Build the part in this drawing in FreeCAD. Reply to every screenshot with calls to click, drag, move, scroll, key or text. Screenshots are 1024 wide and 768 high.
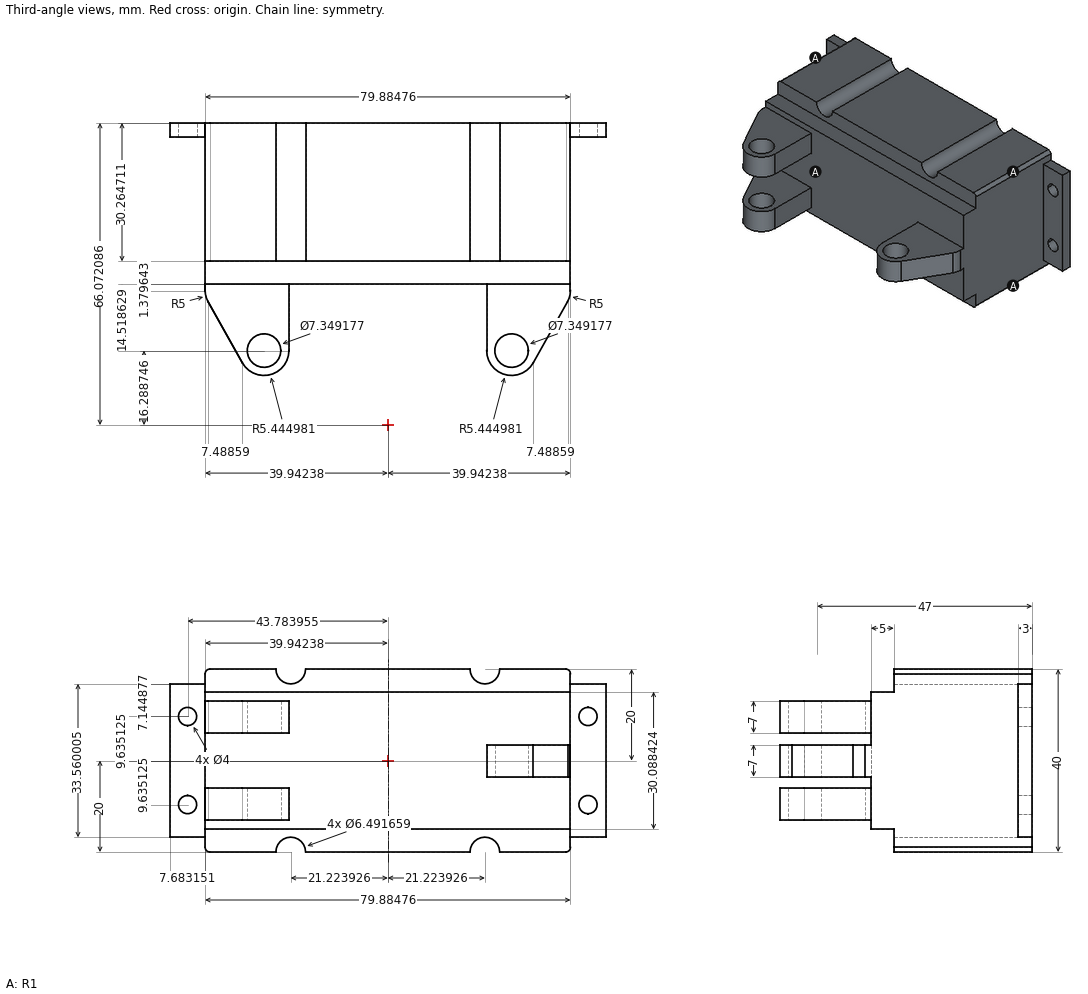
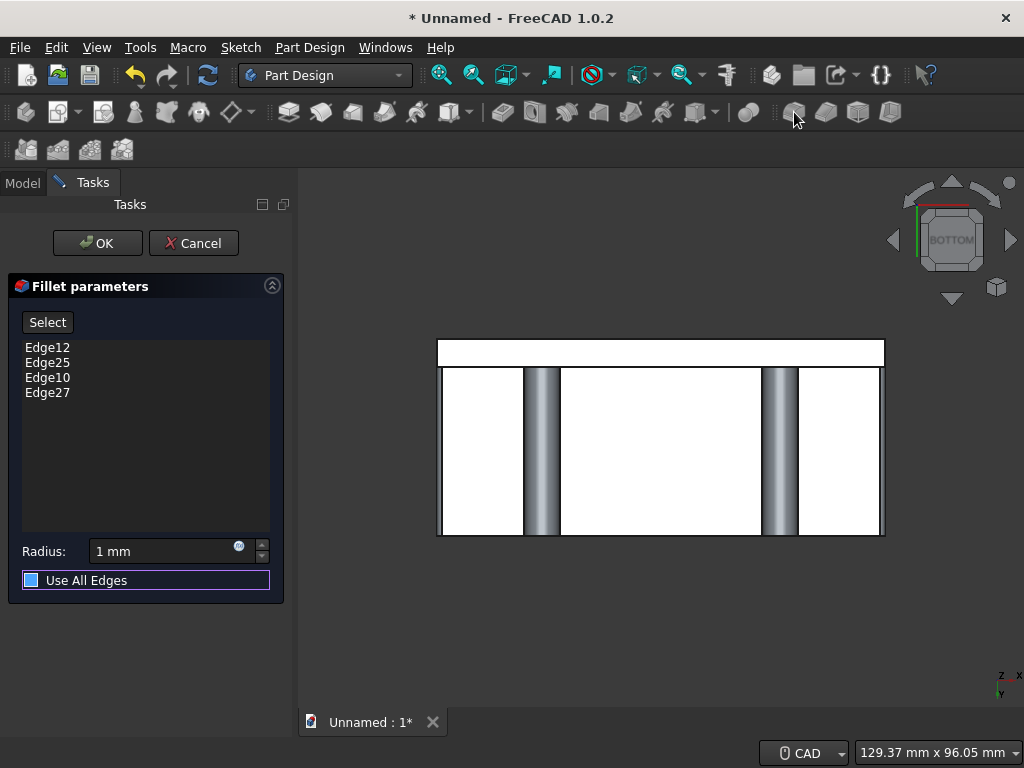
click(98, 243)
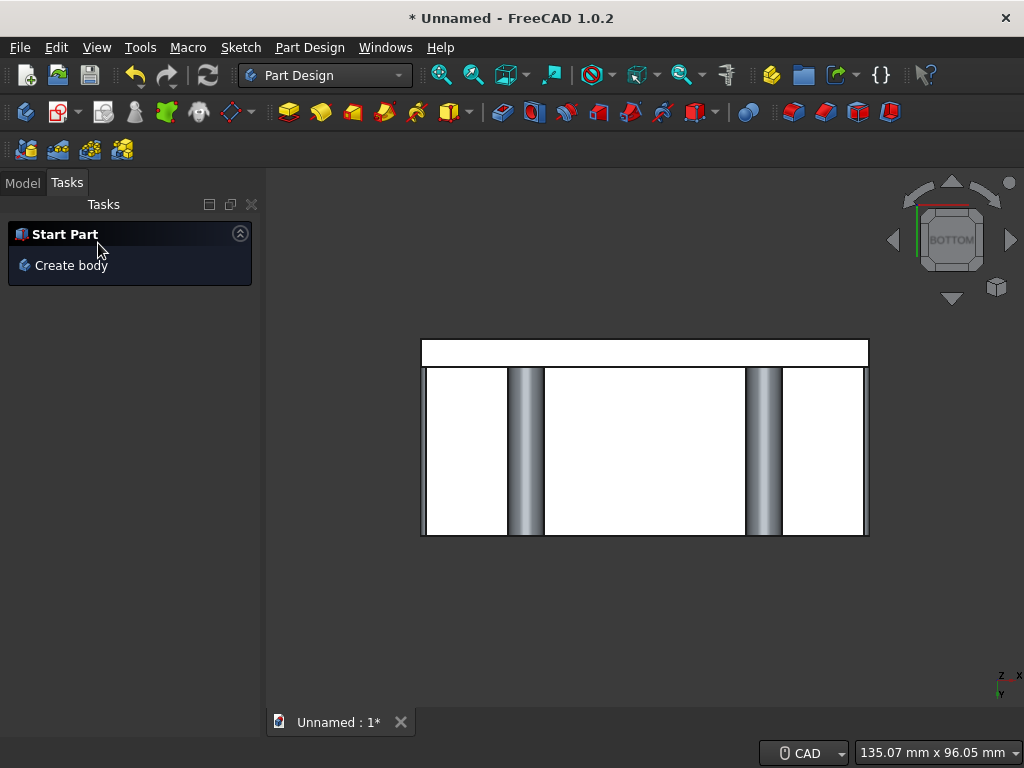
click(23, 182)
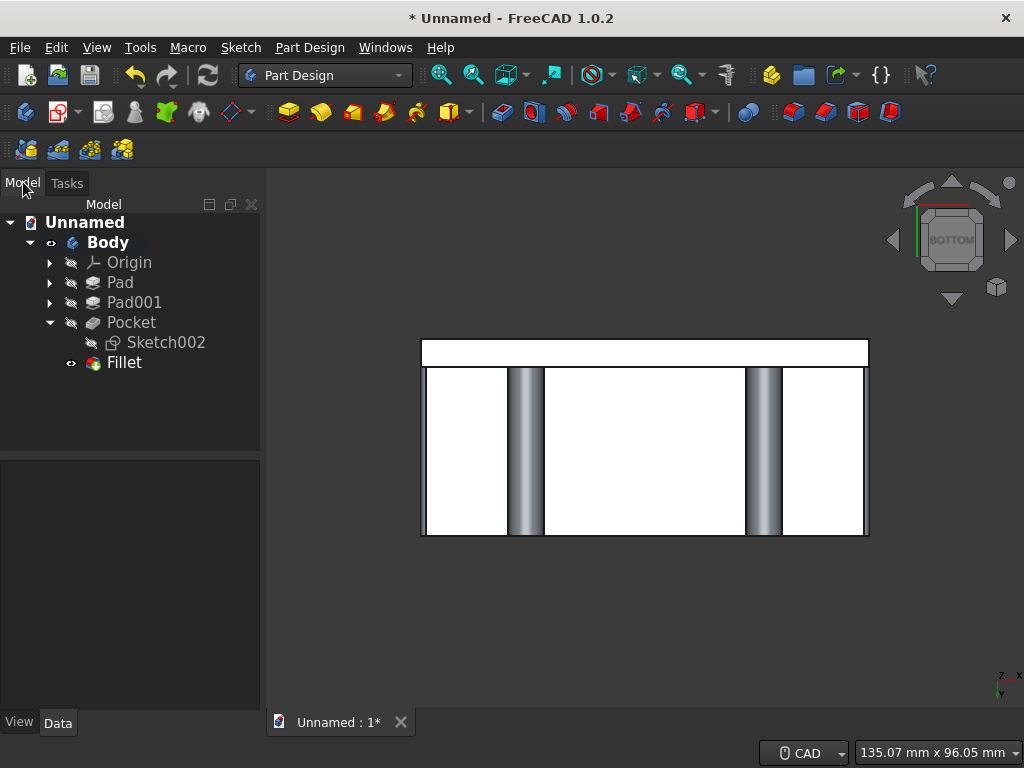
click(50, 263)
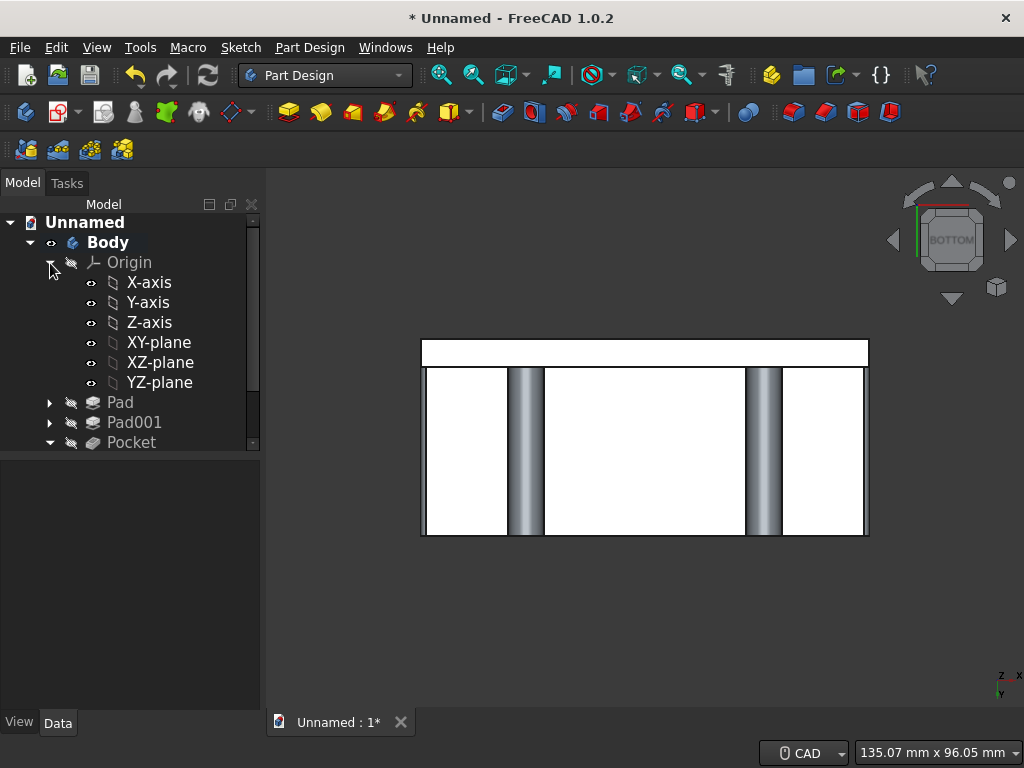
click(136, 343)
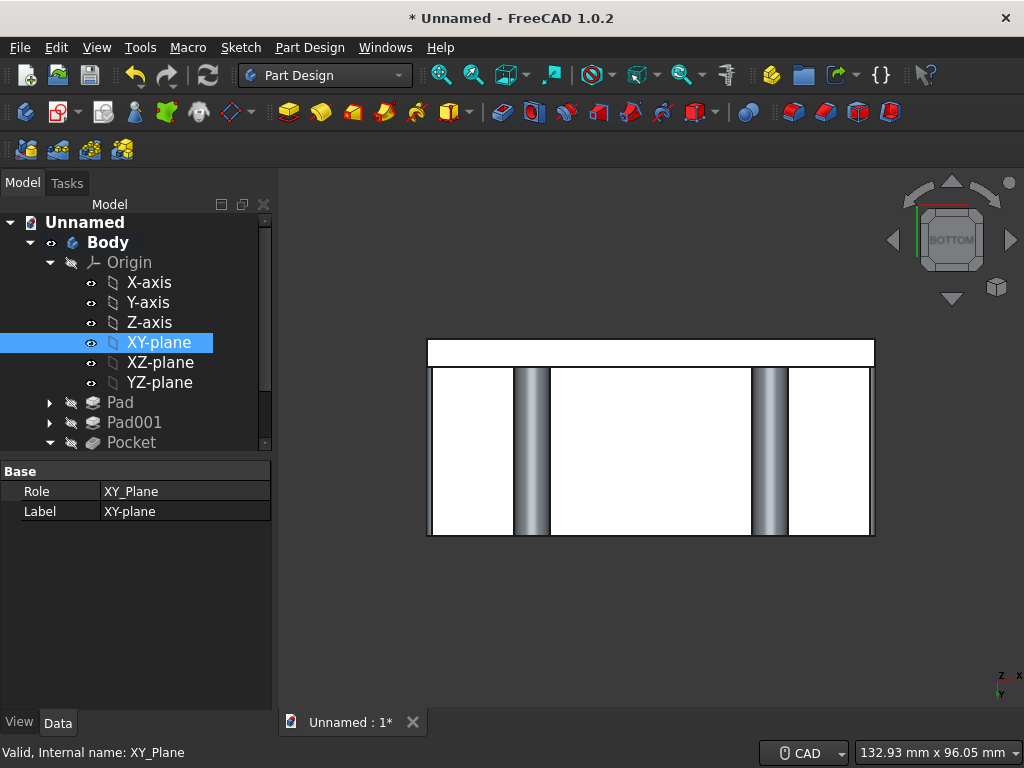
click(232, 112)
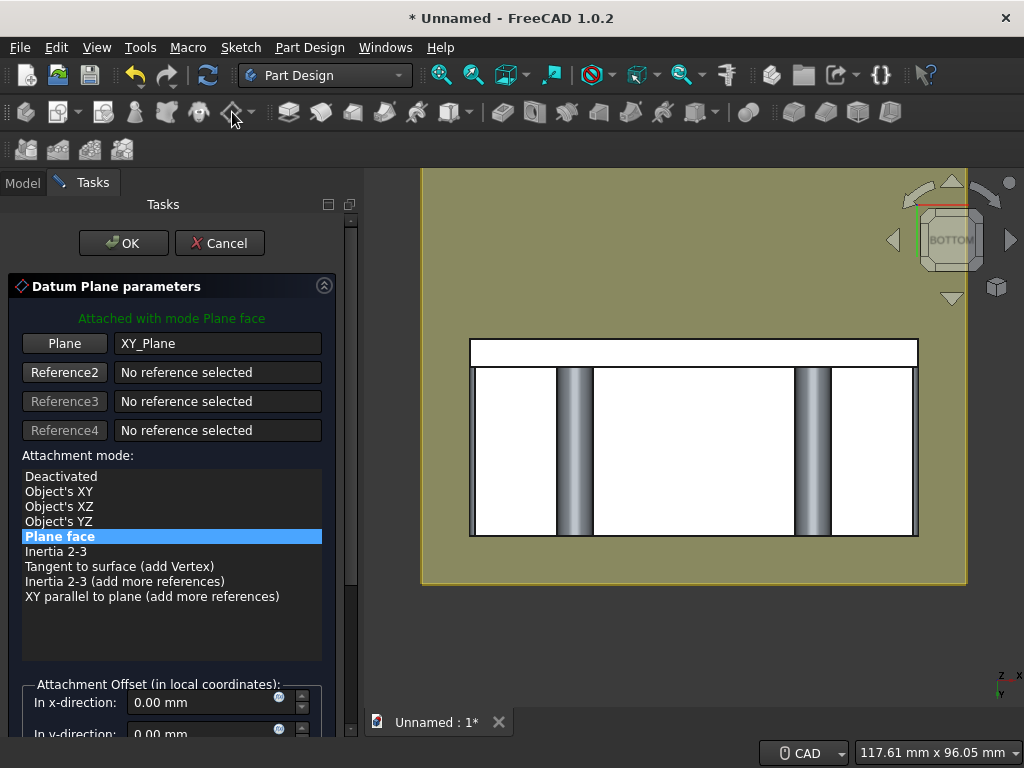
scroll(351, 475, down, 2)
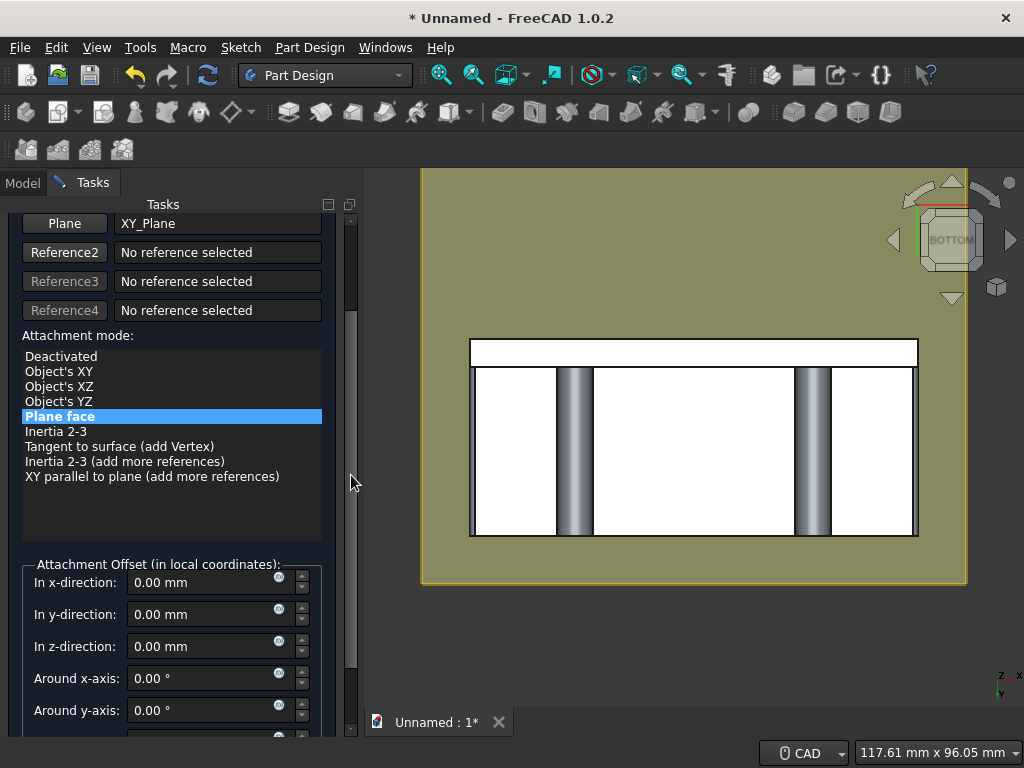
triple_click(210, 646)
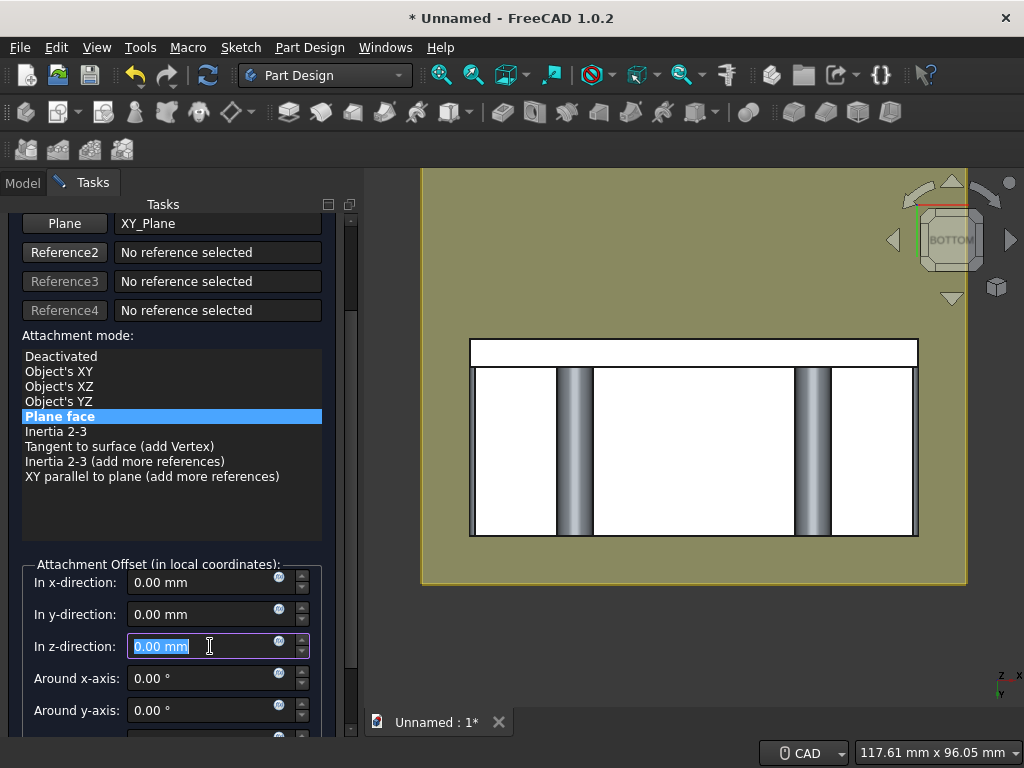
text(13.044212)
key(Tab)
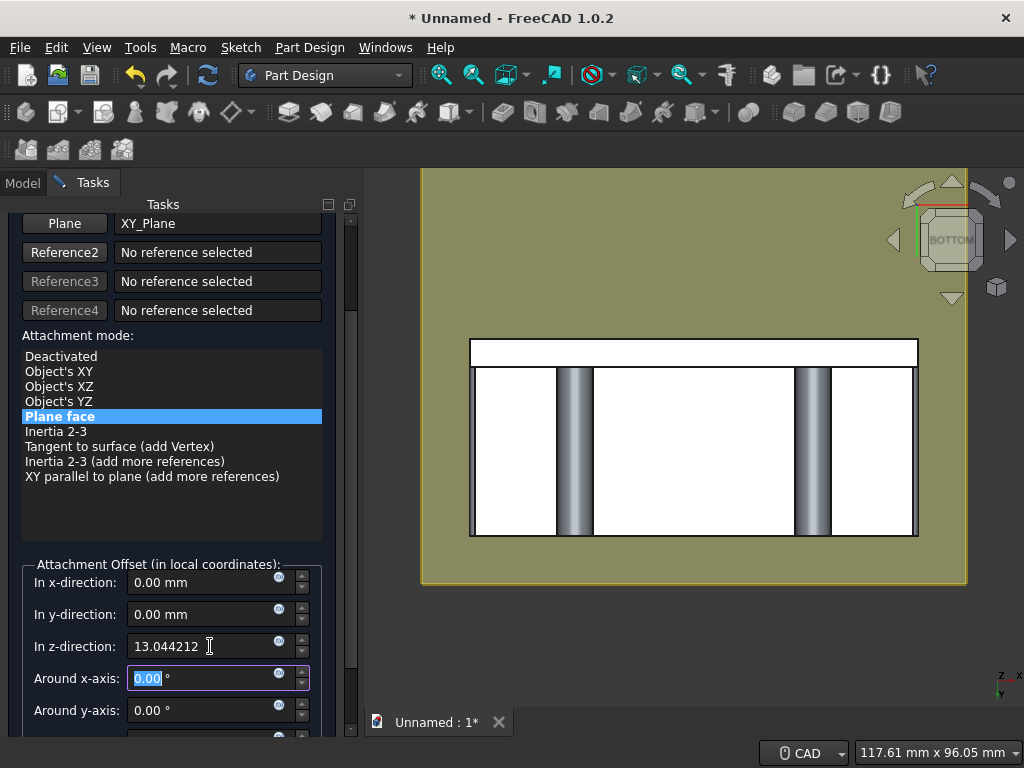
scroll(351, 475, up, 3)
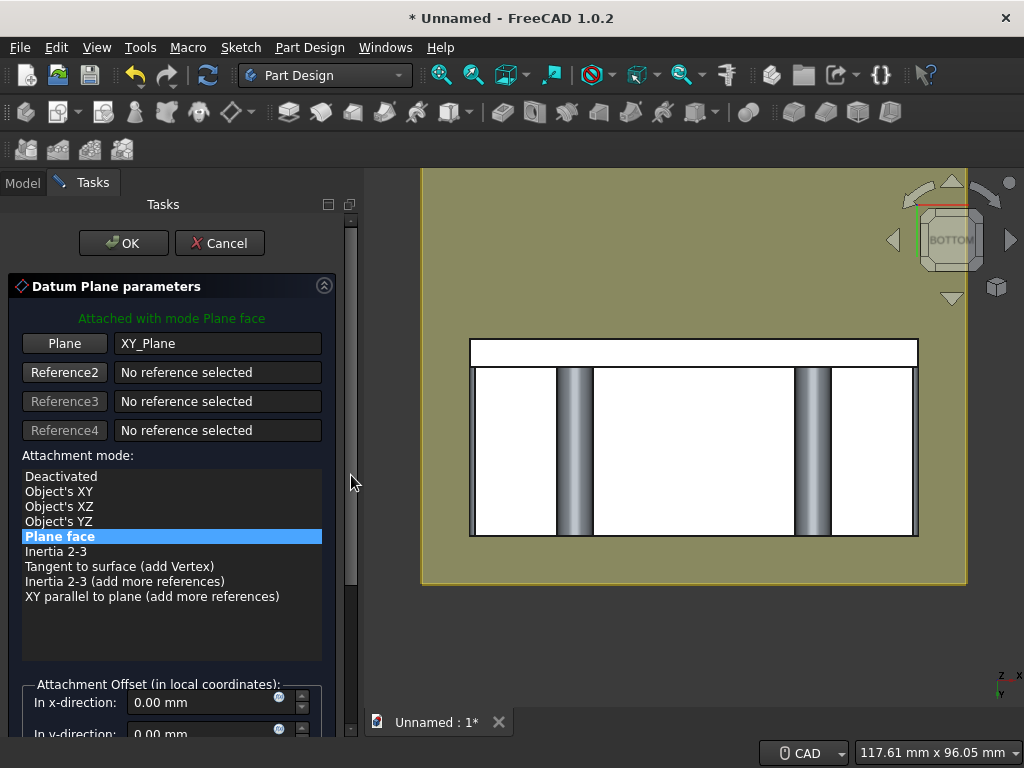
click(124, 243)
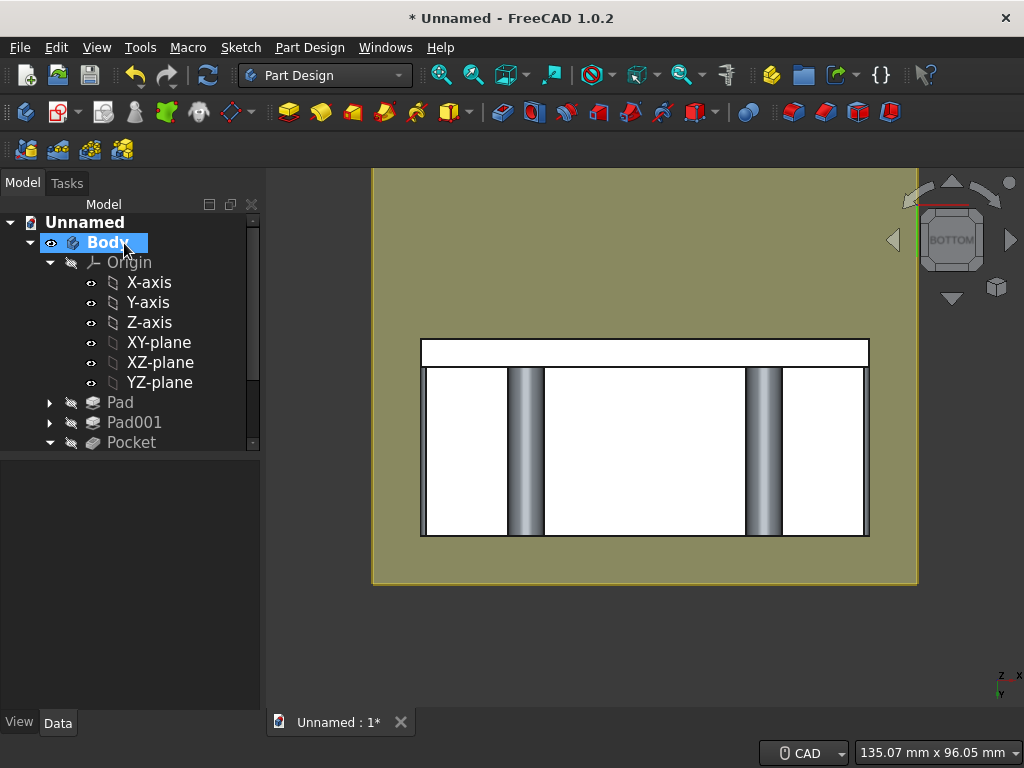
scroll(100, 338, down, 3)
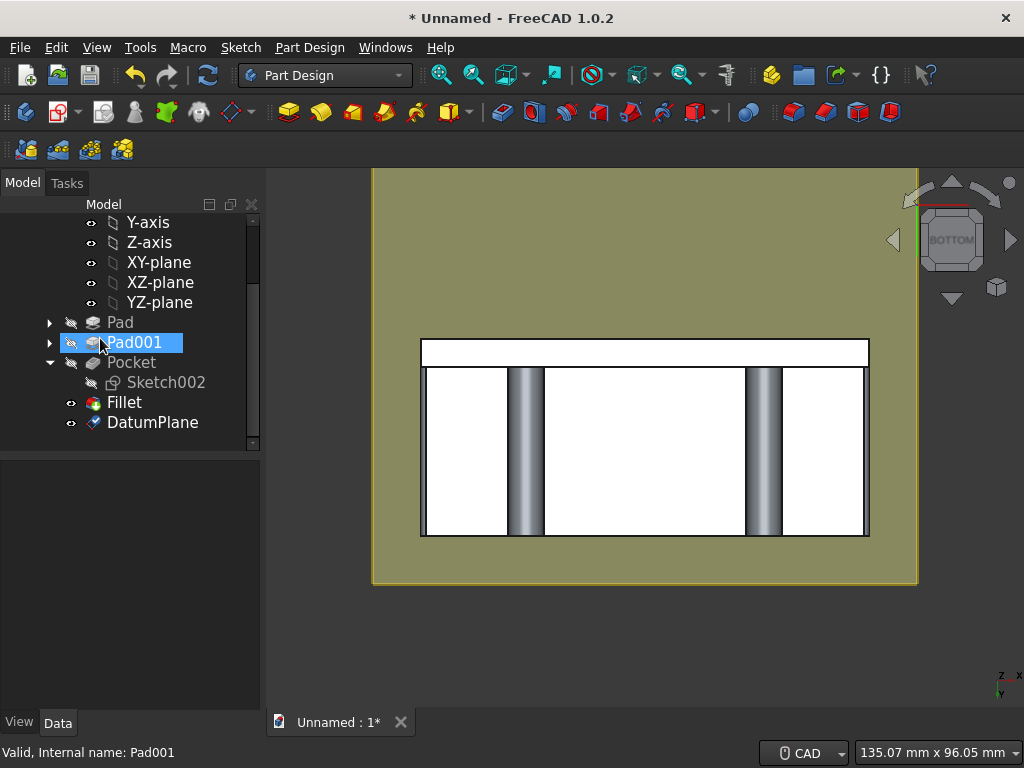
click(116, 423)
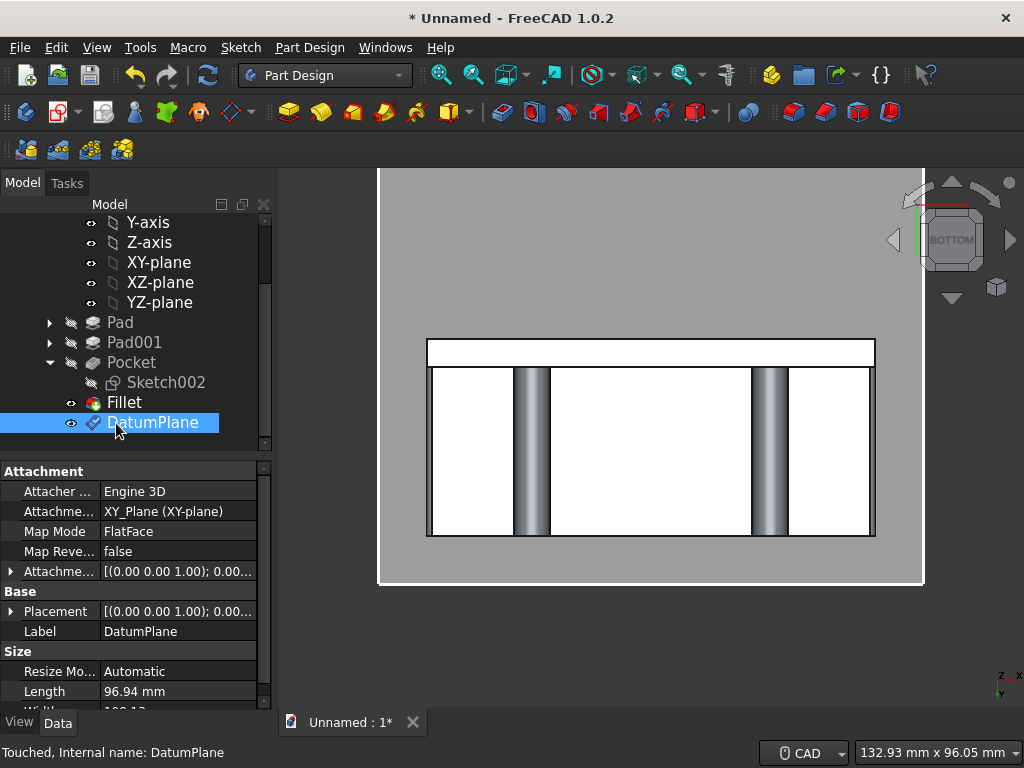
click(58, 112)